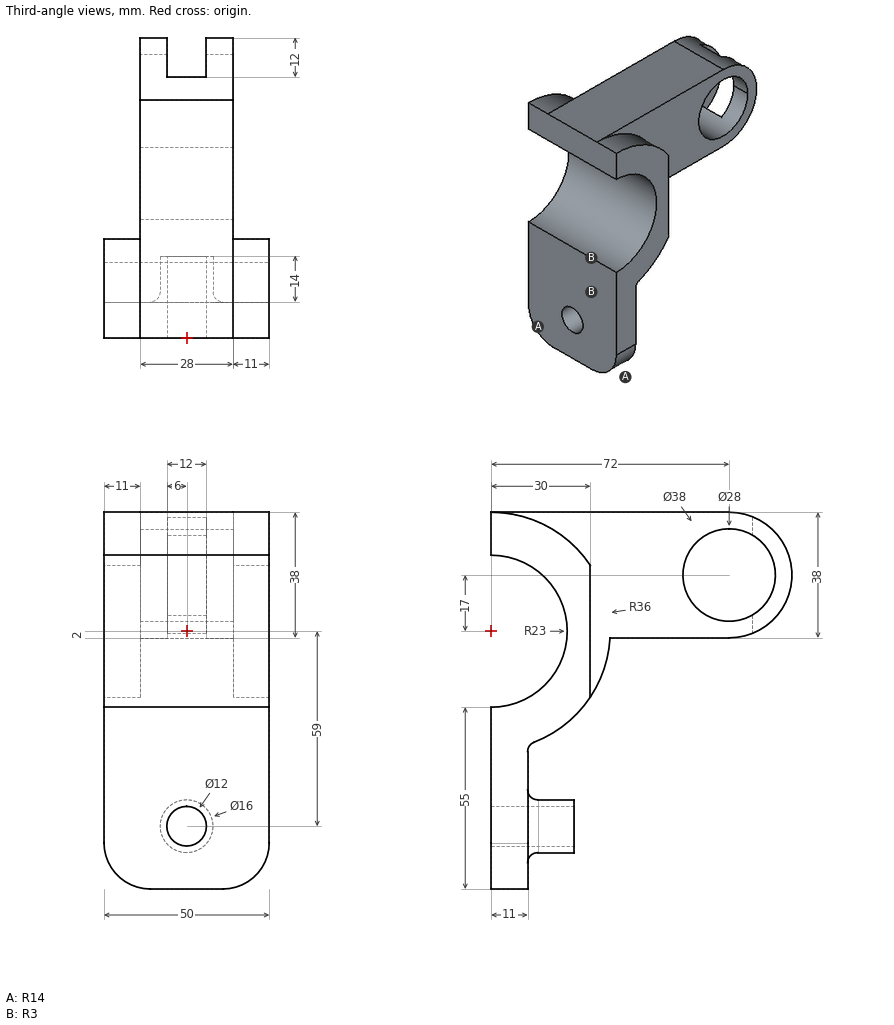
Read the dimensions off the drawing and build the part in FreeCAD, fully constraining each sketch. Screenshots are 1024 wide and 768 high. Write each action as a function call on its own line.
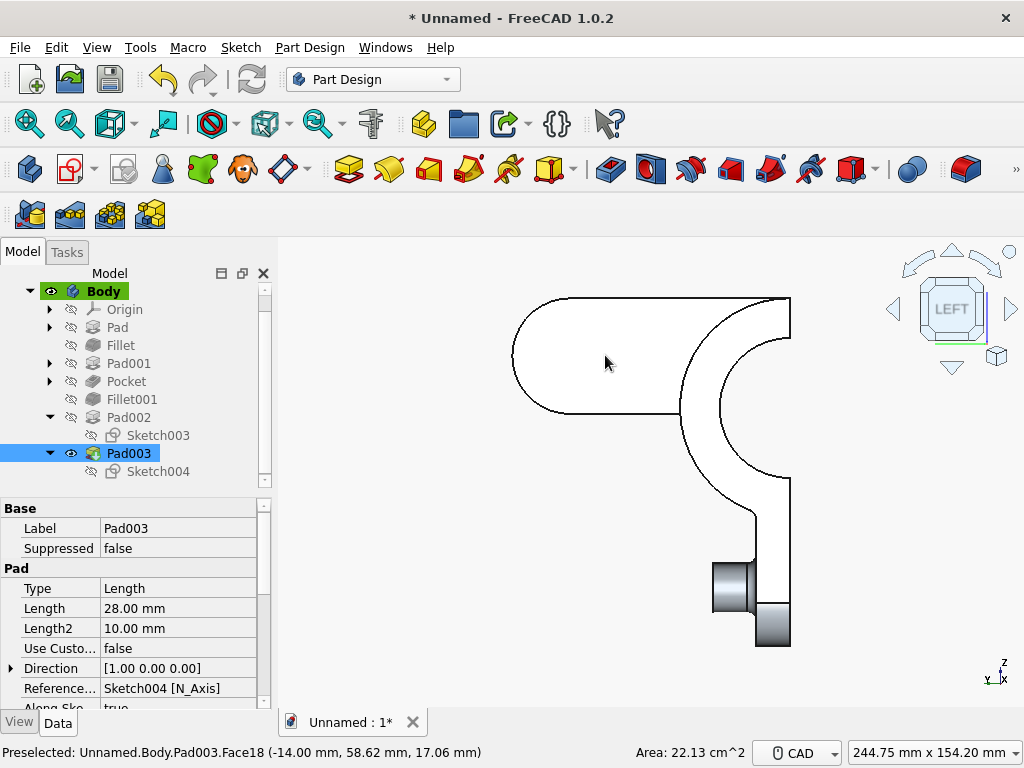
click(70, 170)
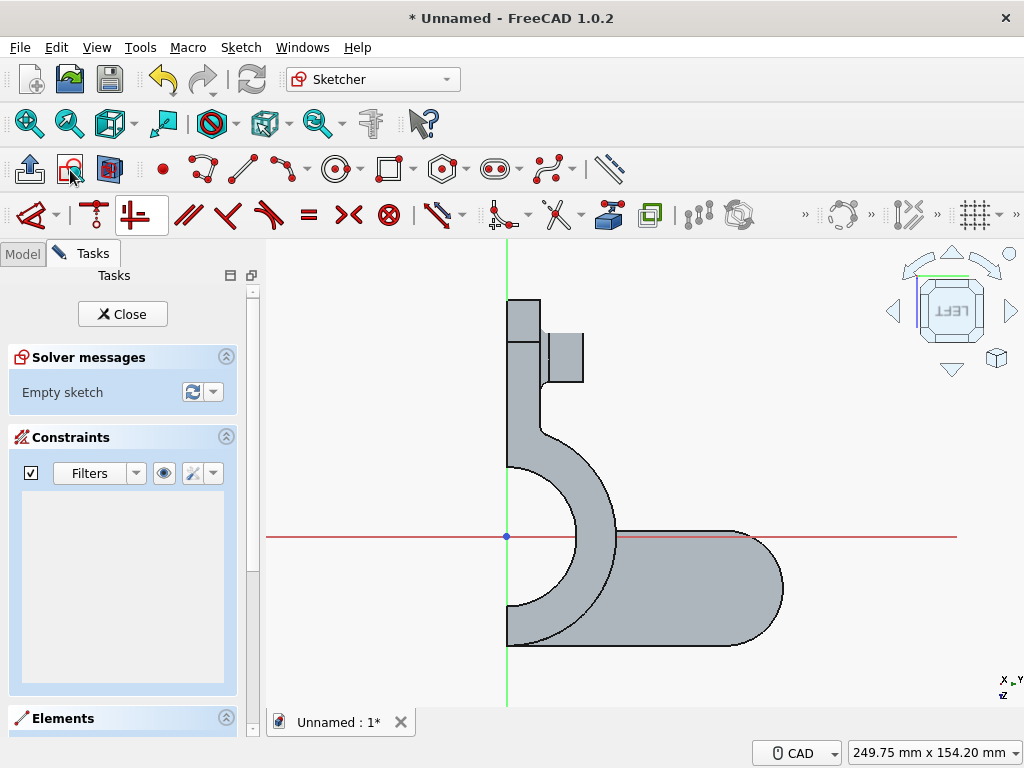
click(110, 170)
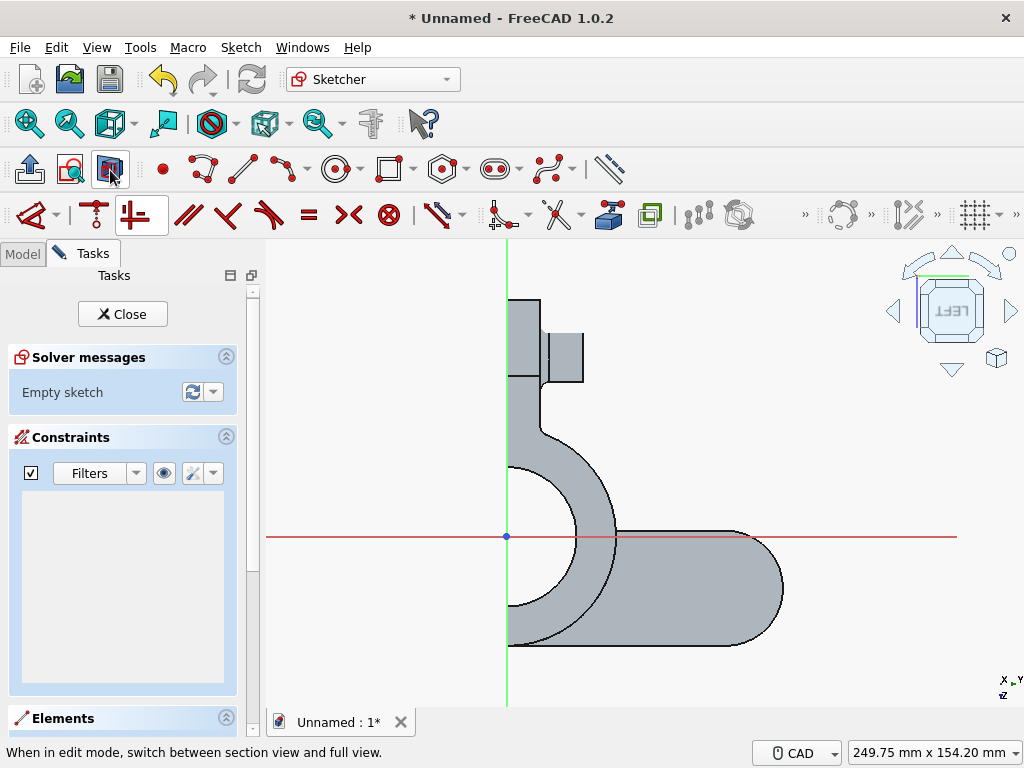
scroll(790, 638, up, 6)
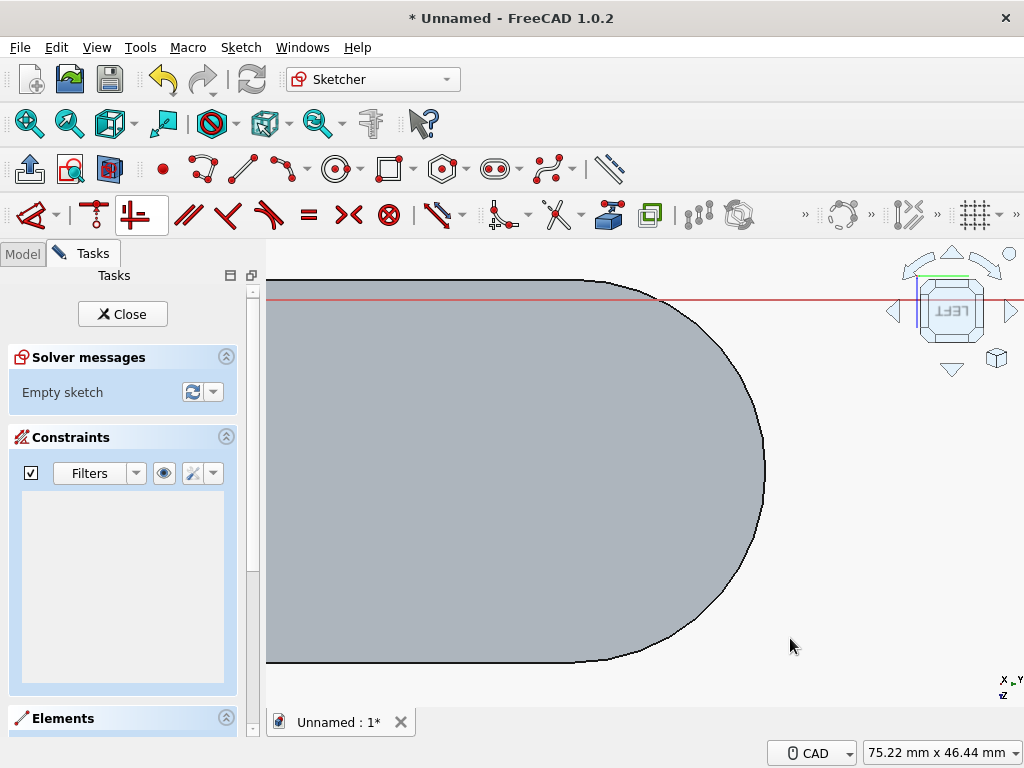
click(336, 170)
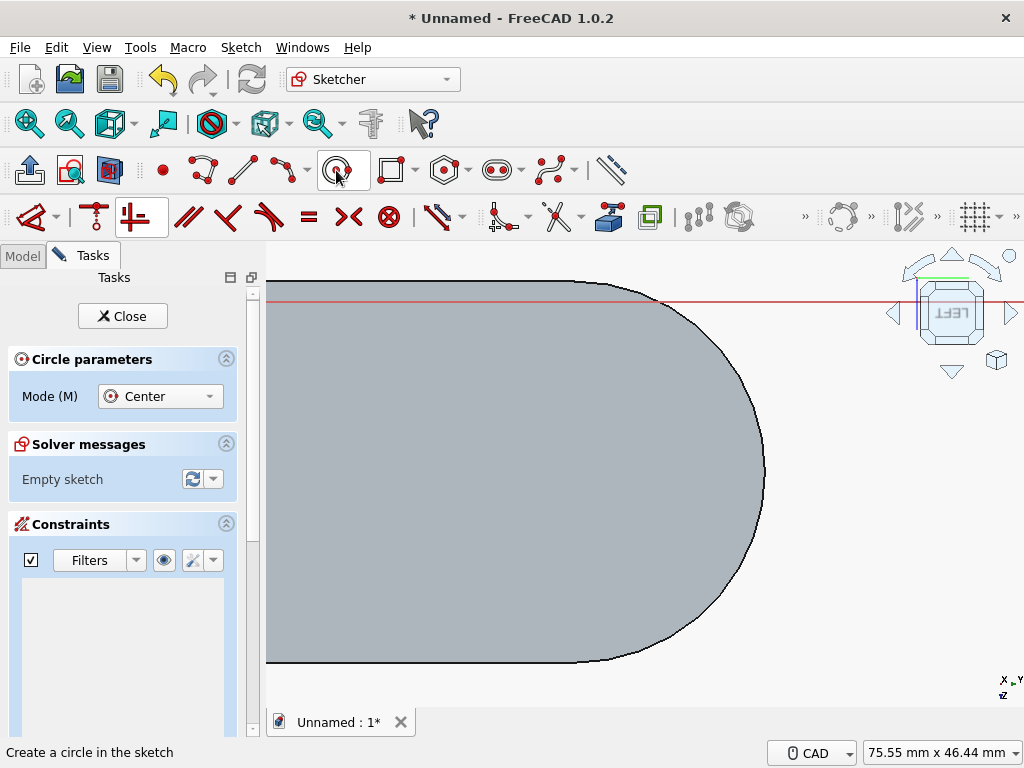
click(574, 472)
move(674, 373)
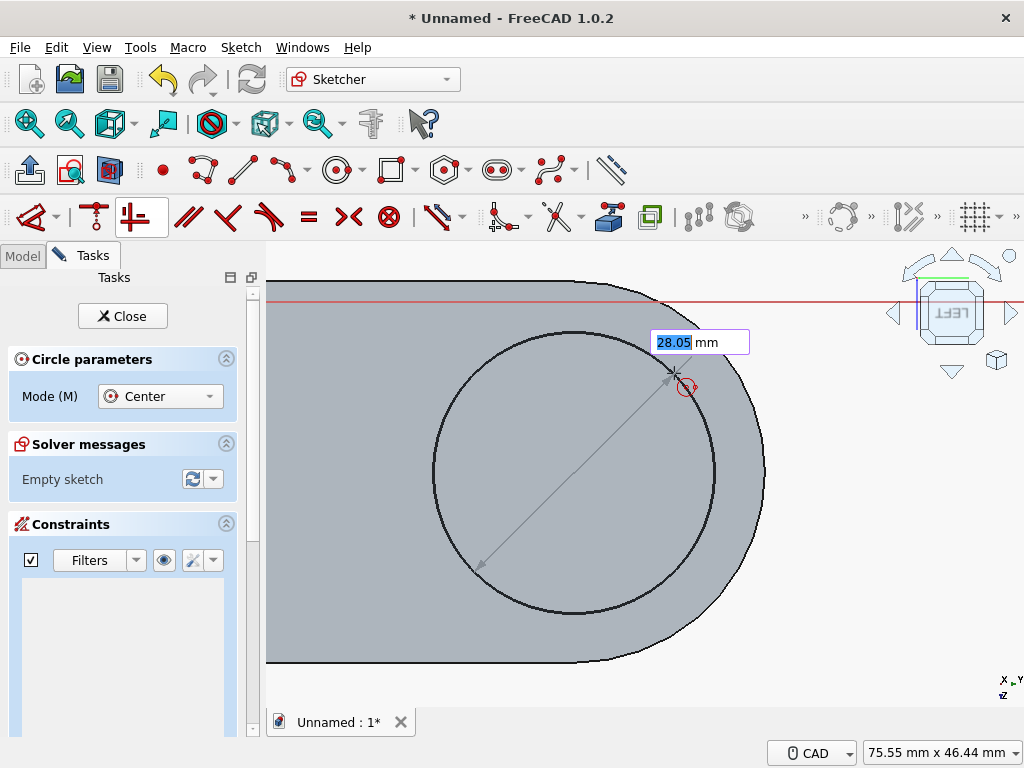
text(28)
key(Return)
key(Escape)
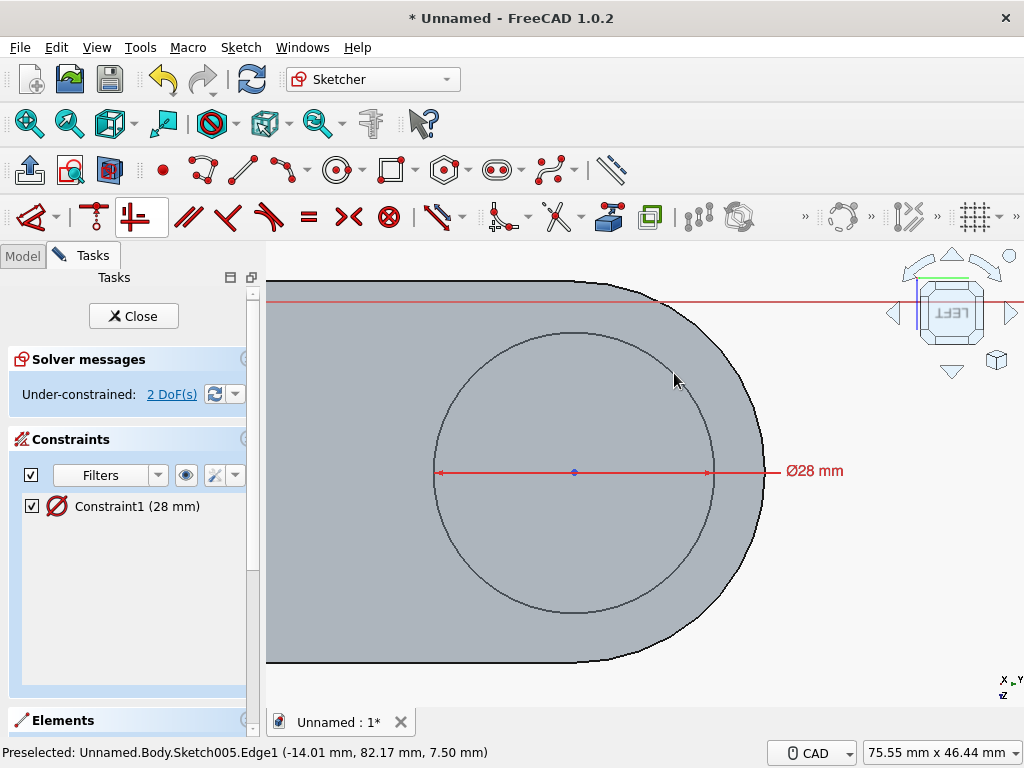
click(32, 218)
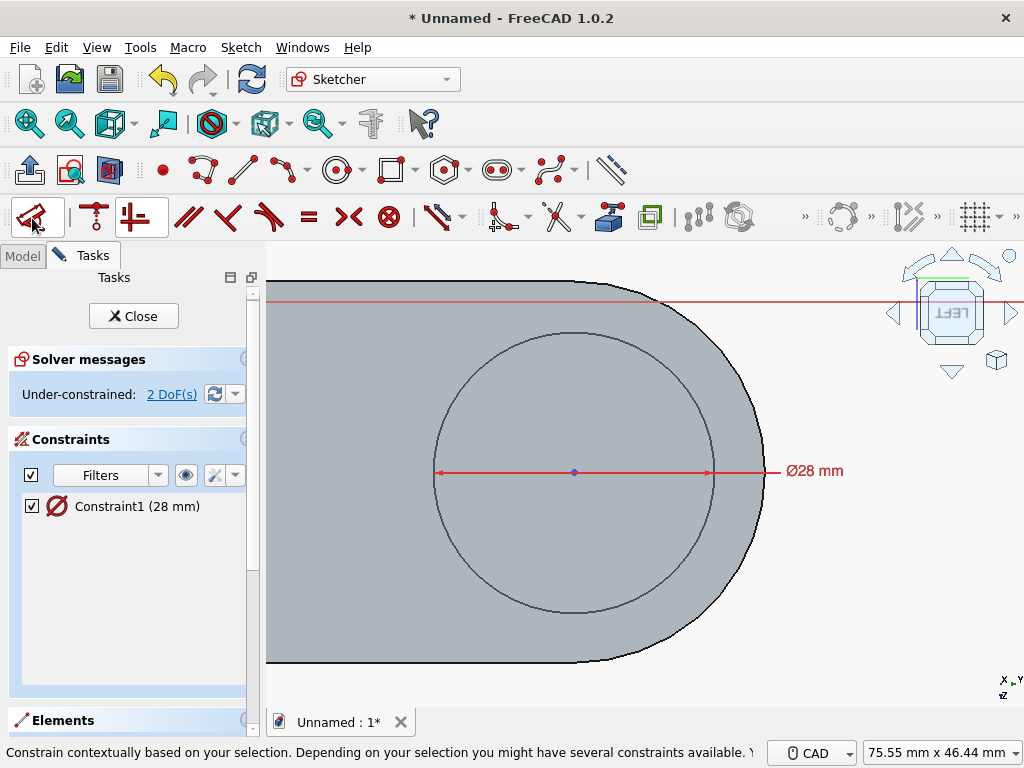
click(574, 473)
click(370, 507)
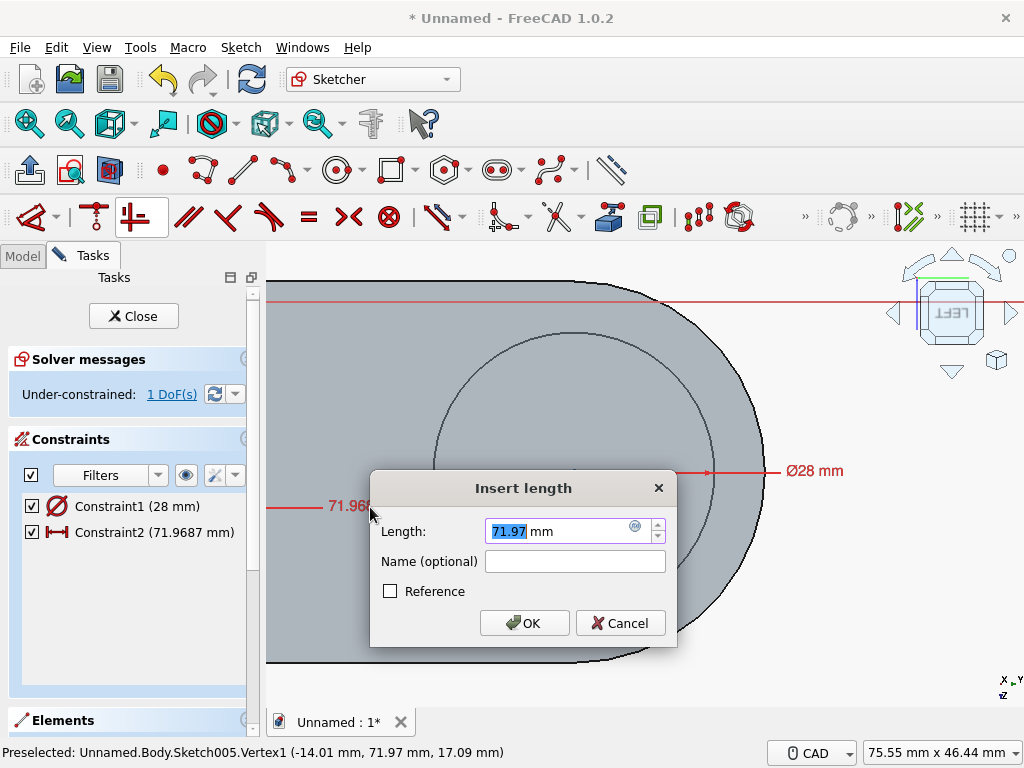
text(72)
key(Return)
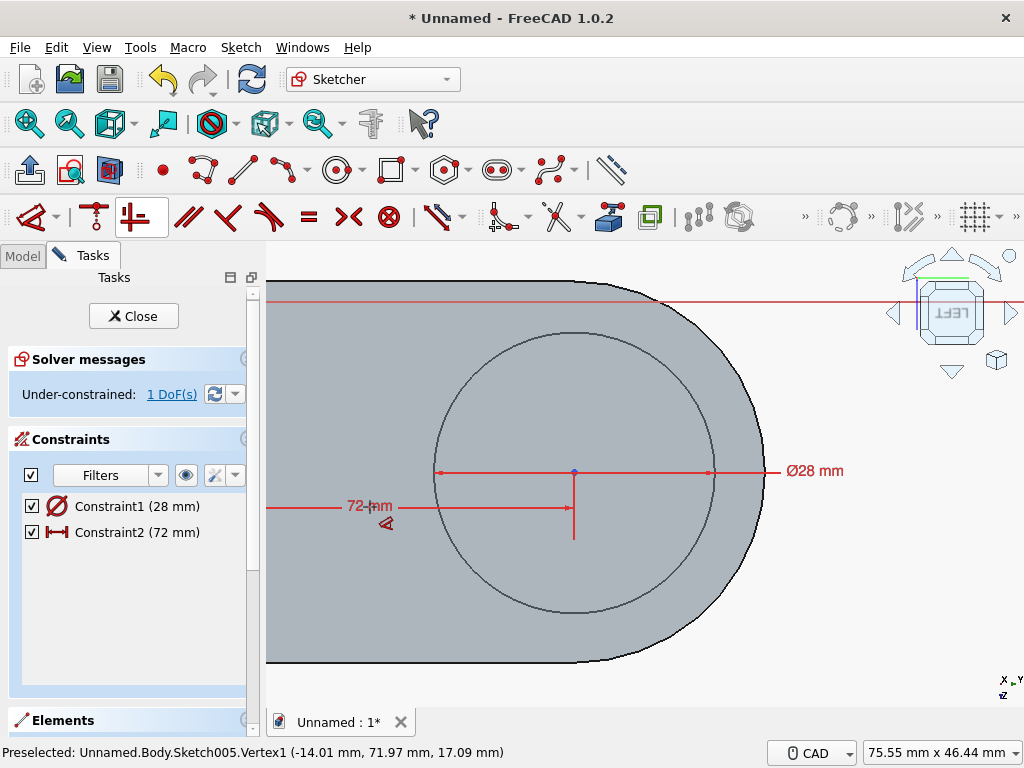
click(574, 473)
click(608, 387)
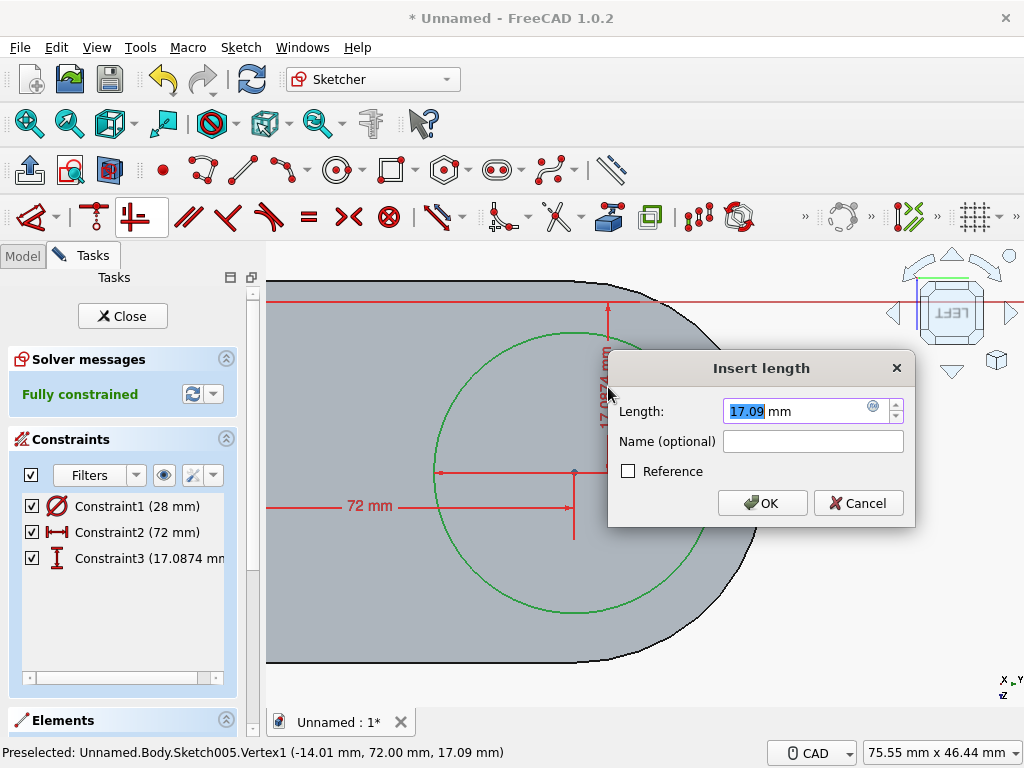
text(17)
key(Return)
key(Escape)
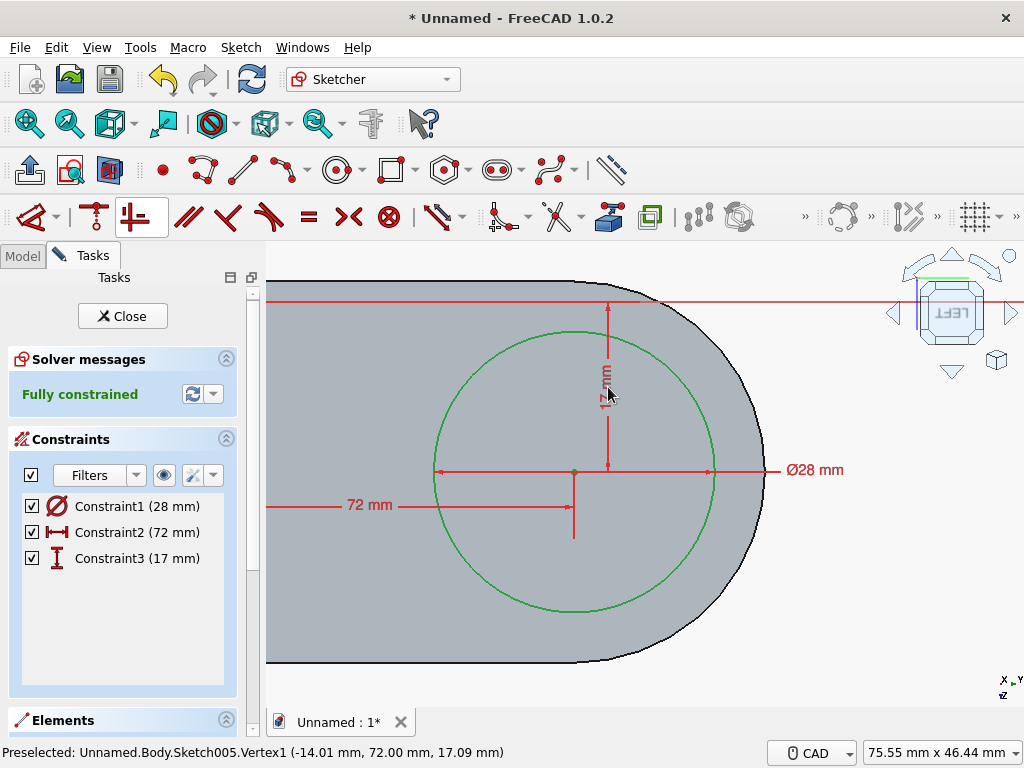
click(123, 316)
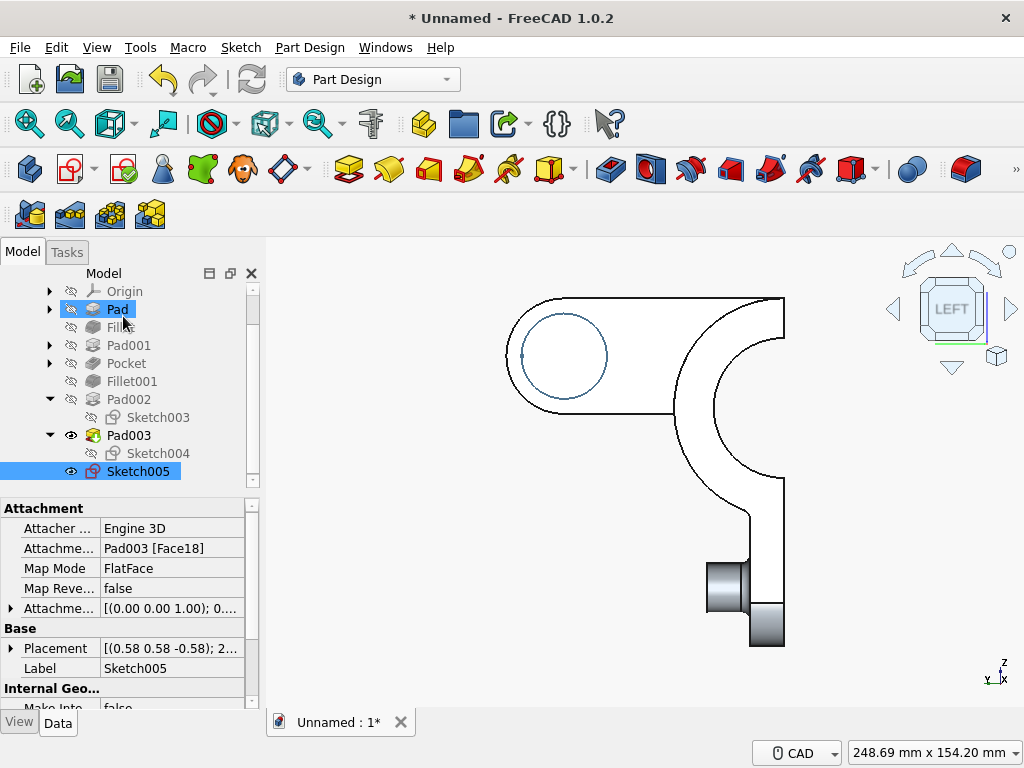
click(612, 170)